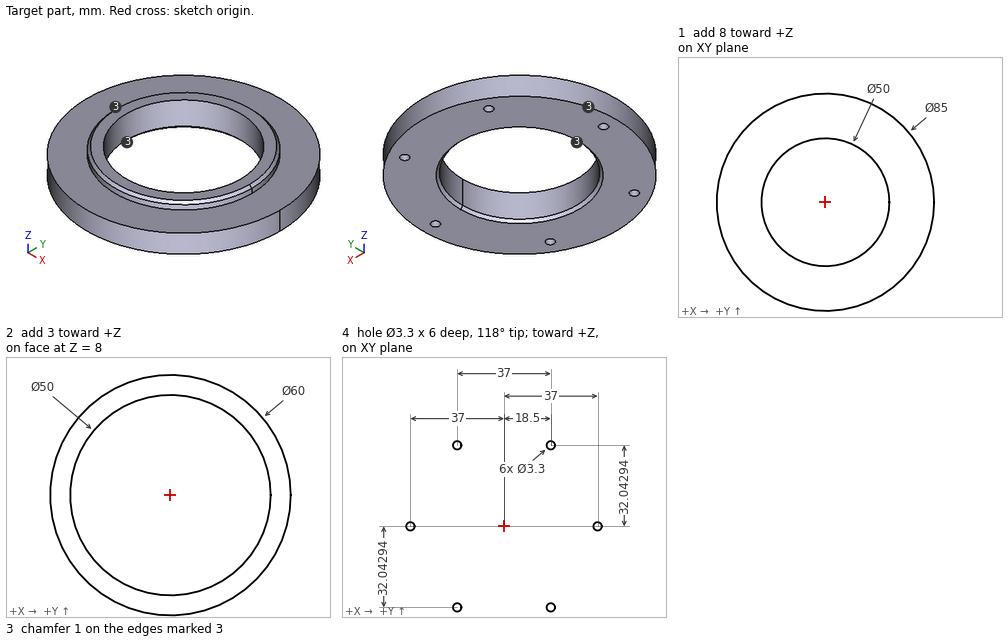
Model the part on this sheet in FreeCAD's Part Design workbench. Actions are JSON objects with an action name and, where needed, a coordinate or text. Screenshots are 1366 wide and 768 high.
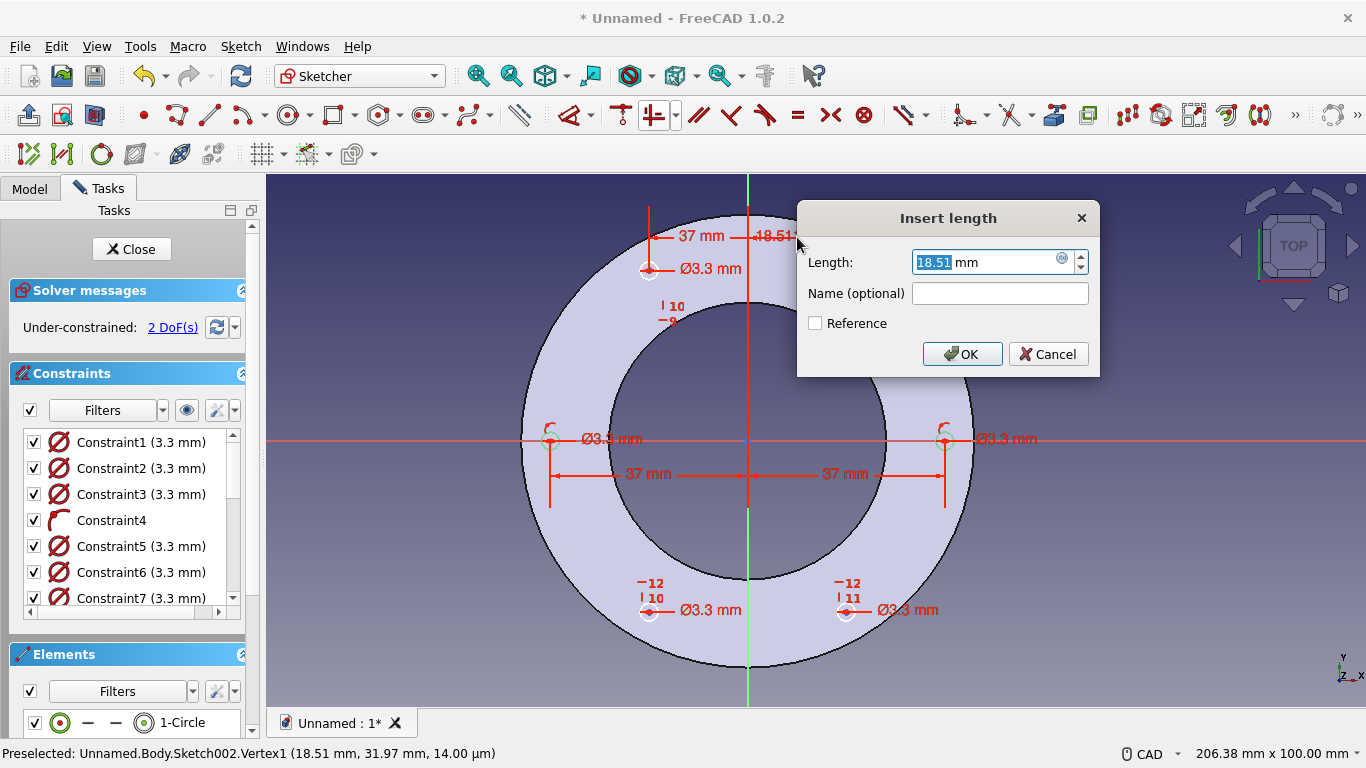
{"action": "type", "text": "18.5"}
{"action": "key", "text": "Return"}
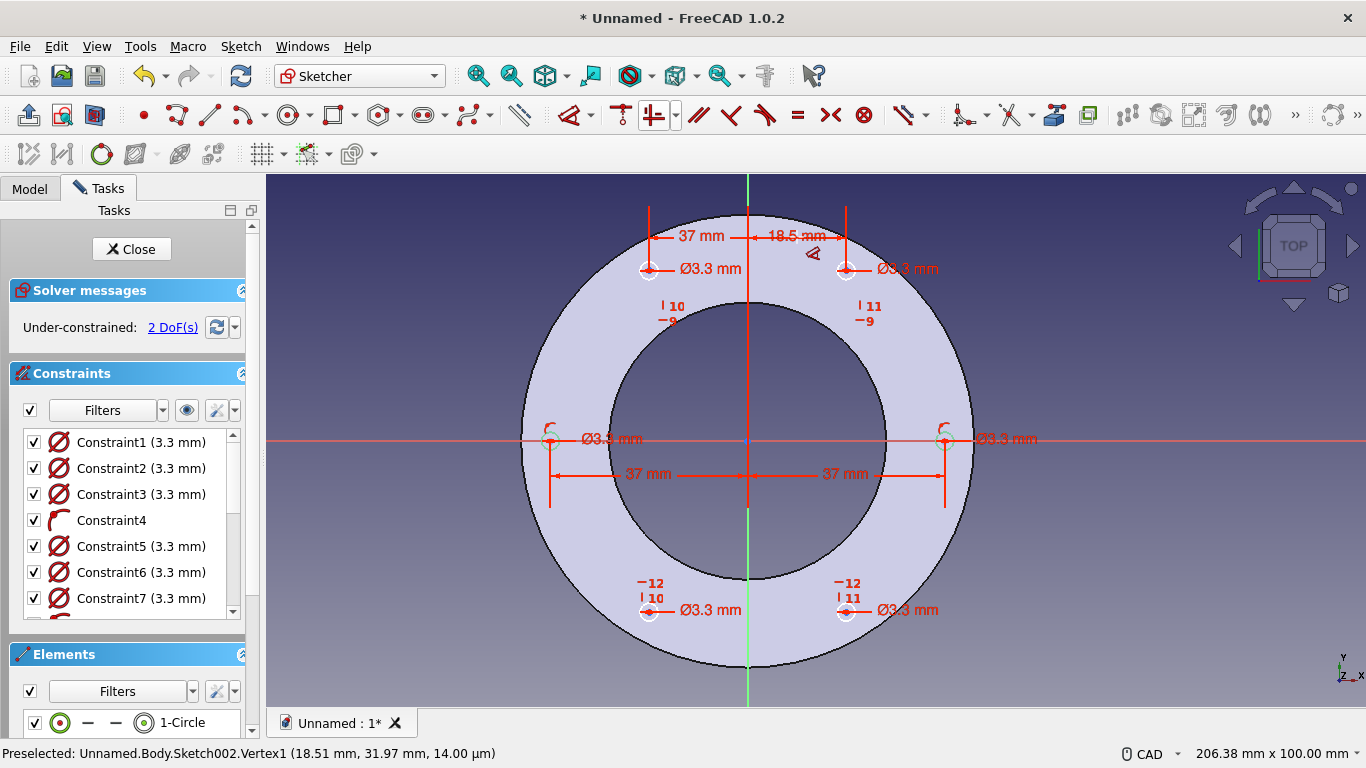
{"action": "left_click", "coordinate": [846, 271]}
{"action": "left_click", "coordinate": [880, 356]}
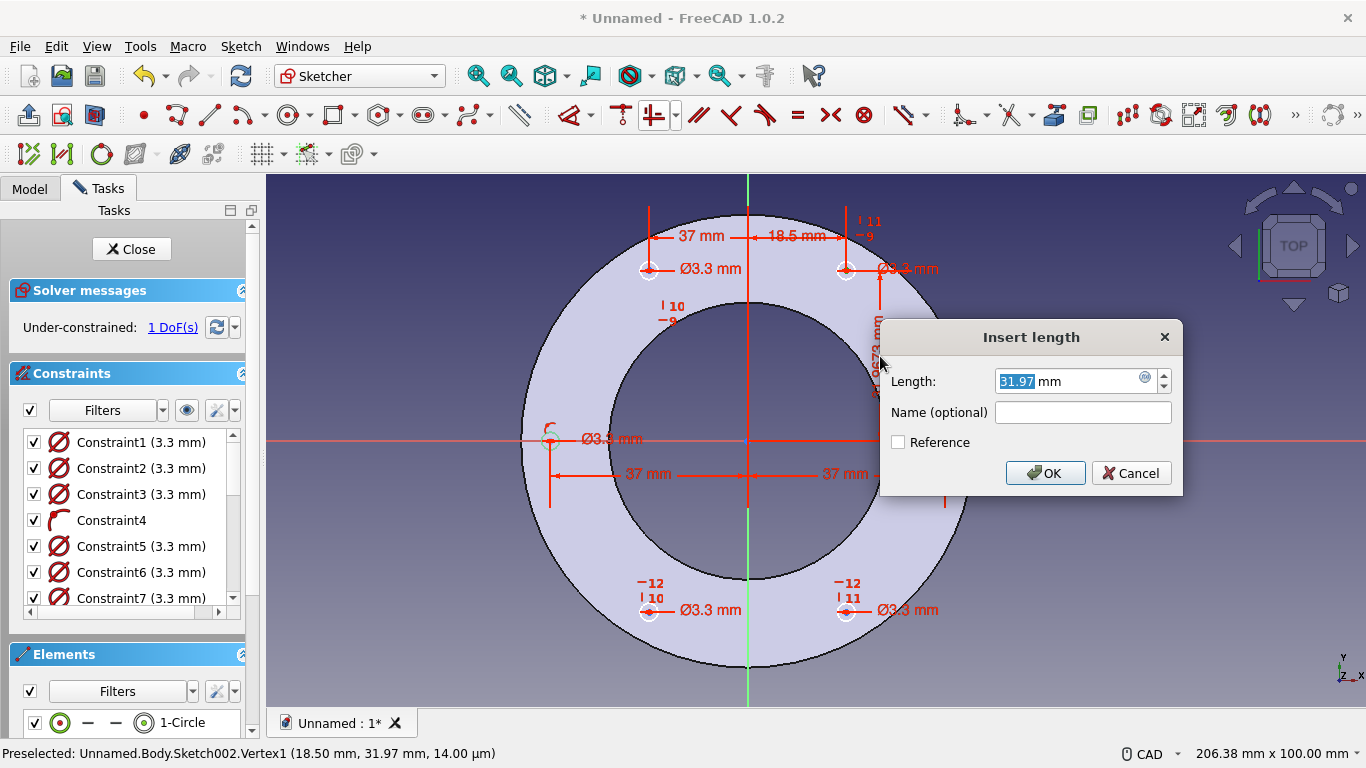
{"action": "type", "text": "32.04294"}
{"action": "key", "text": "Return"}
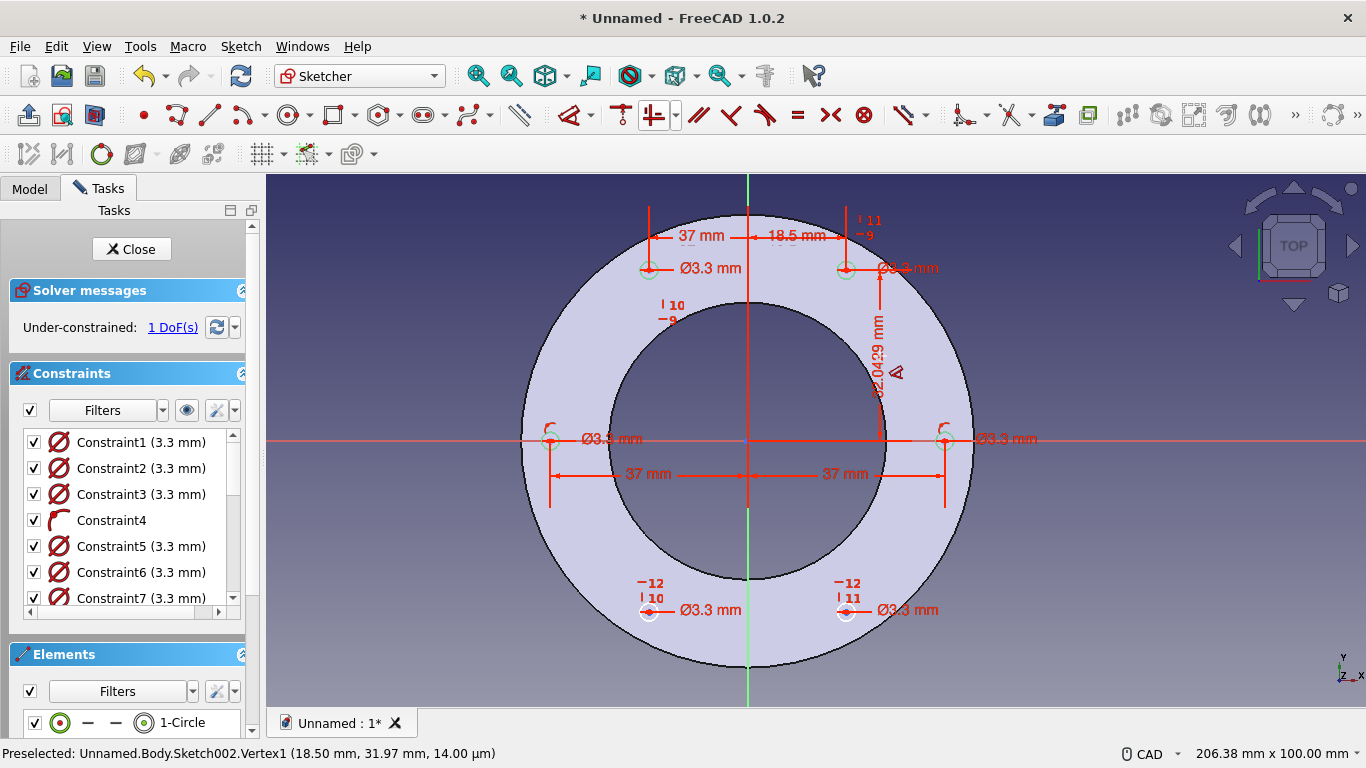
{"action": "left_click", "coordinate": [649, 612]}
{"action": "left_click", "coordinate": [615, 527]}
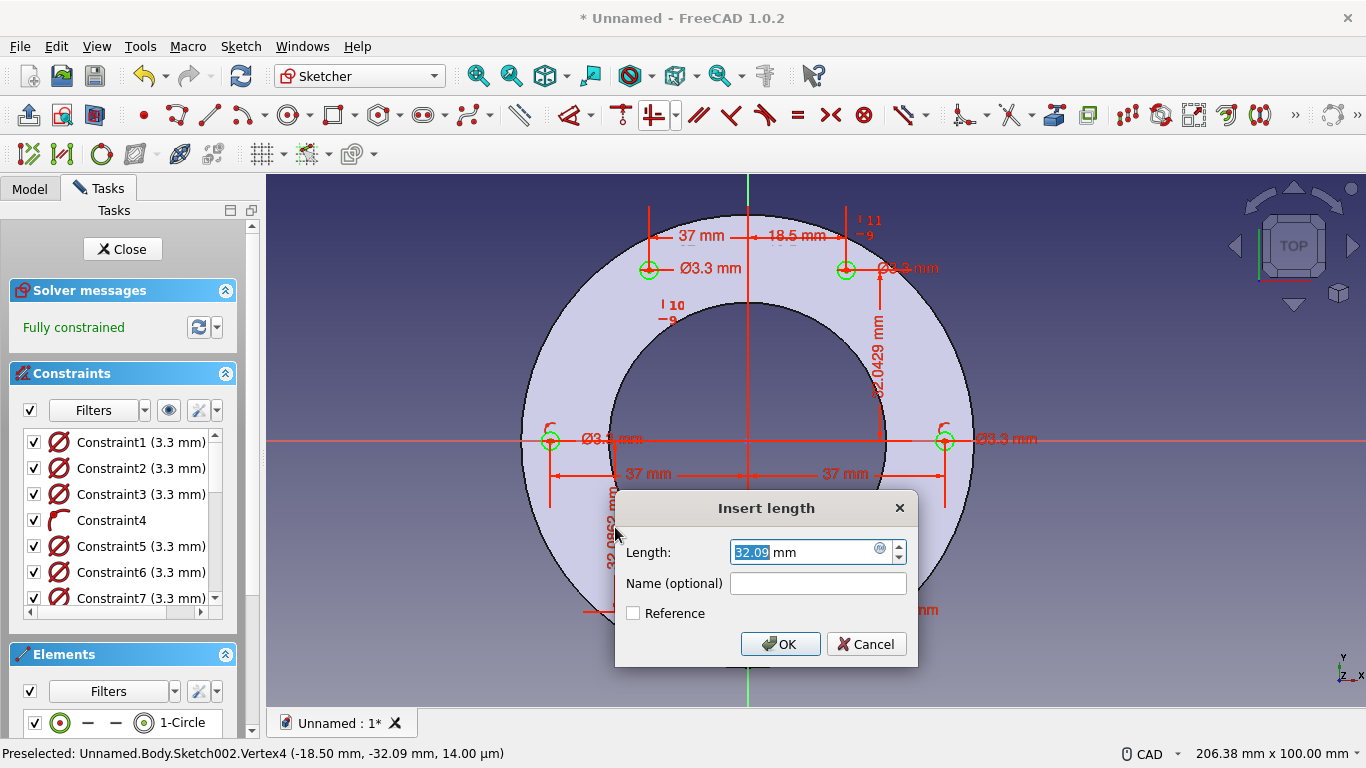
{"action": "type", "text": "32.04294"}
{"action": "key", "text": "Return"}
{"action": "key", "text": "Escape"}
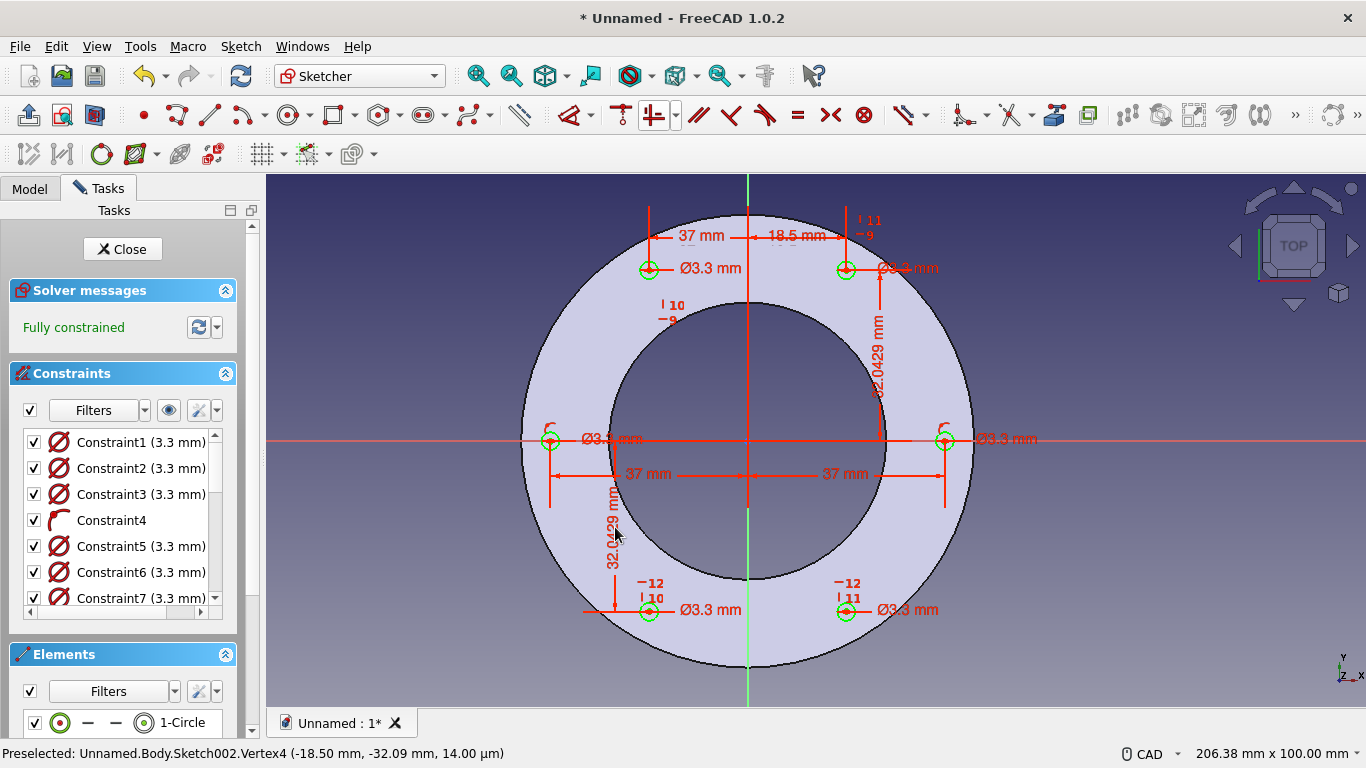
{"action": "left_click", "coordinate": [123, 249]}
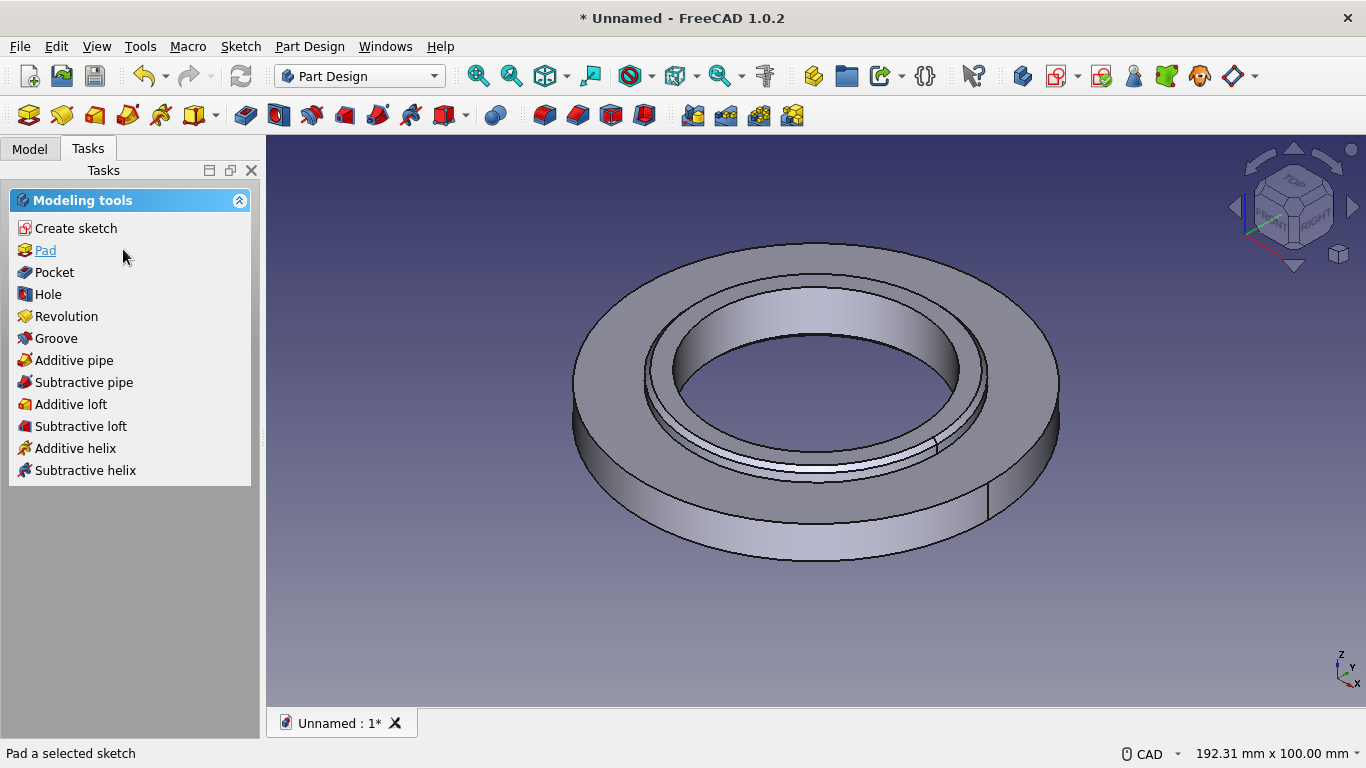
{"action": "left_click", "coordinate": [279, 116]}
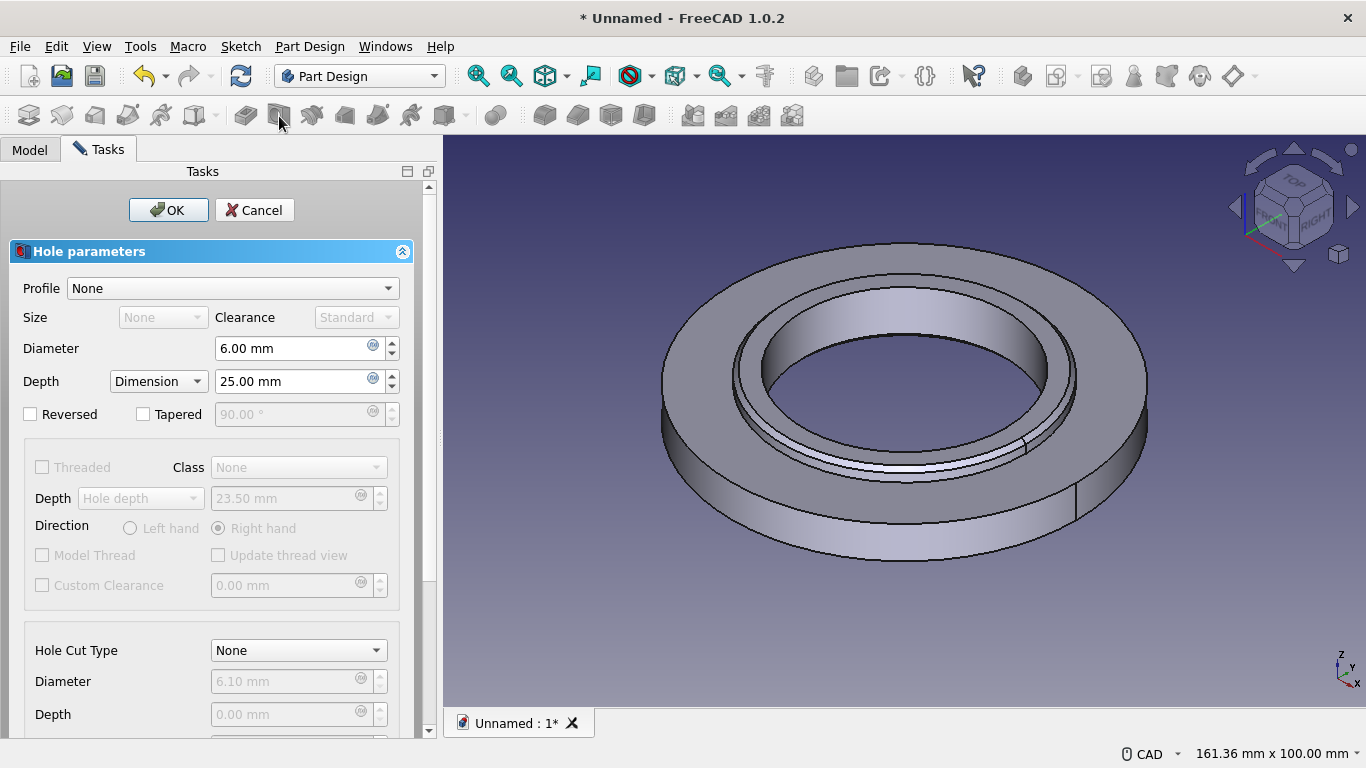
{"action": "triple_click", "coordinate": [300, 348]}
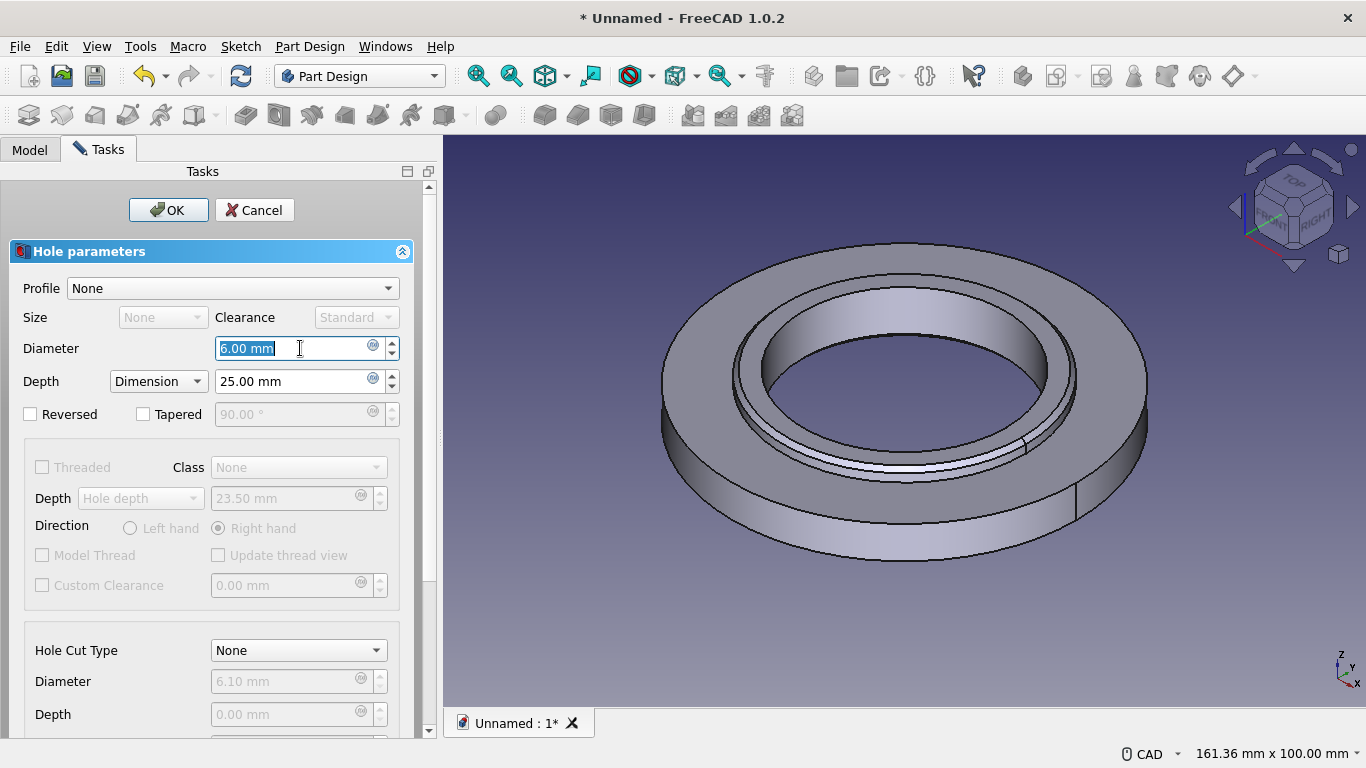
{"action": "type", "text": "3.3"}
{"action": "key", "text": "Tab"}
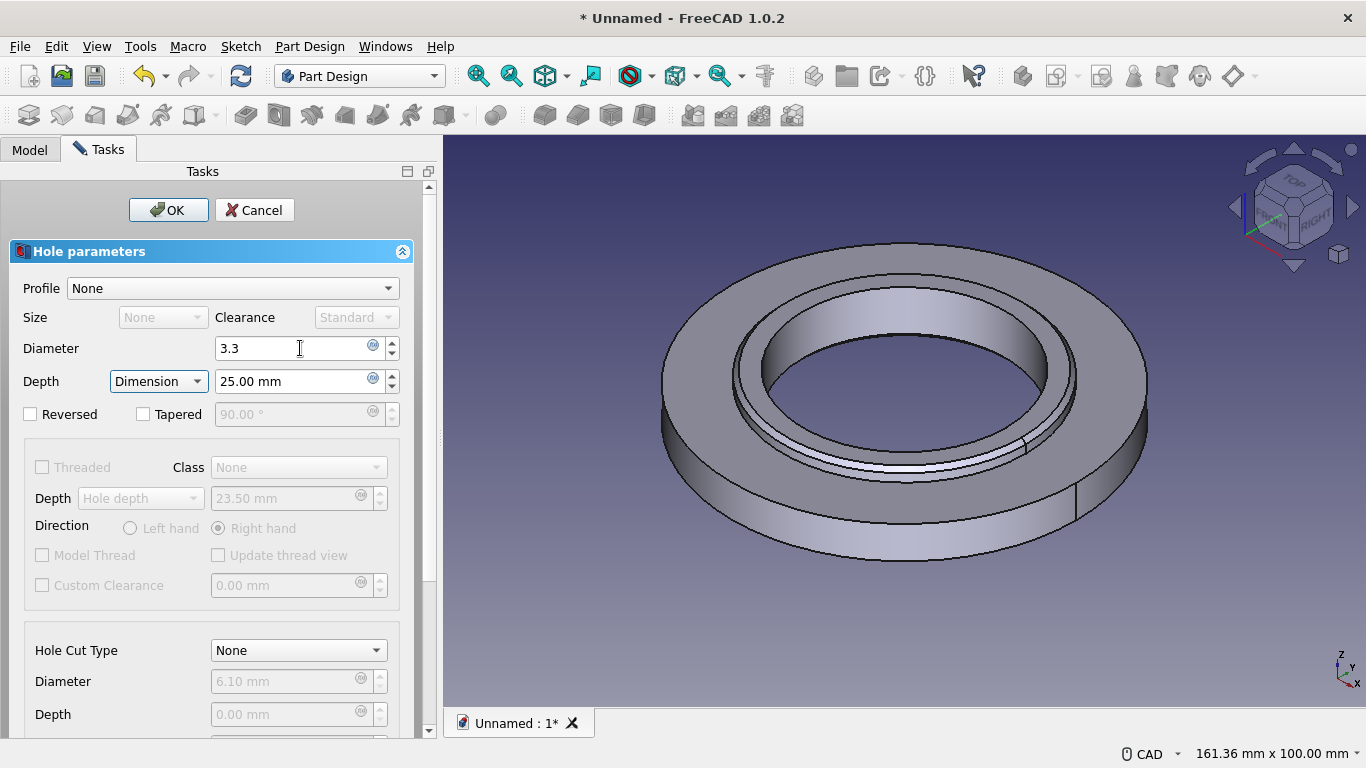
{"action": "triple_click", "coordinate": [300, 382]}